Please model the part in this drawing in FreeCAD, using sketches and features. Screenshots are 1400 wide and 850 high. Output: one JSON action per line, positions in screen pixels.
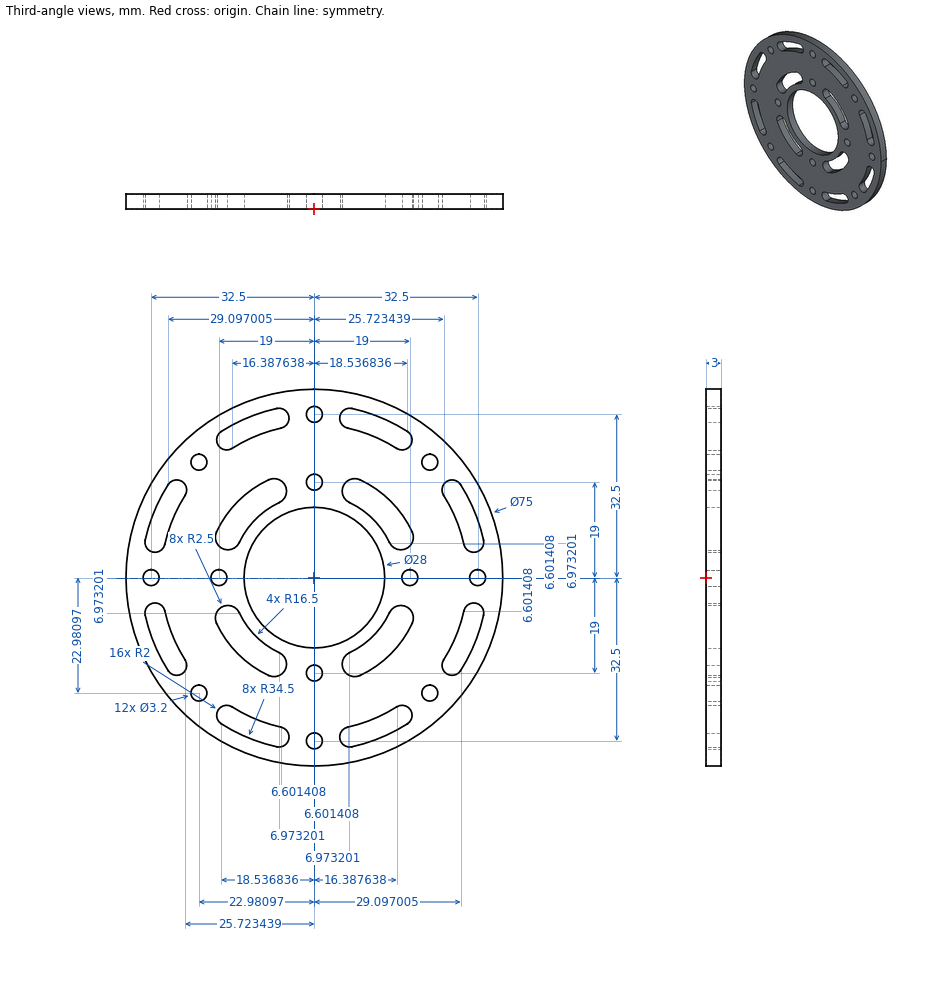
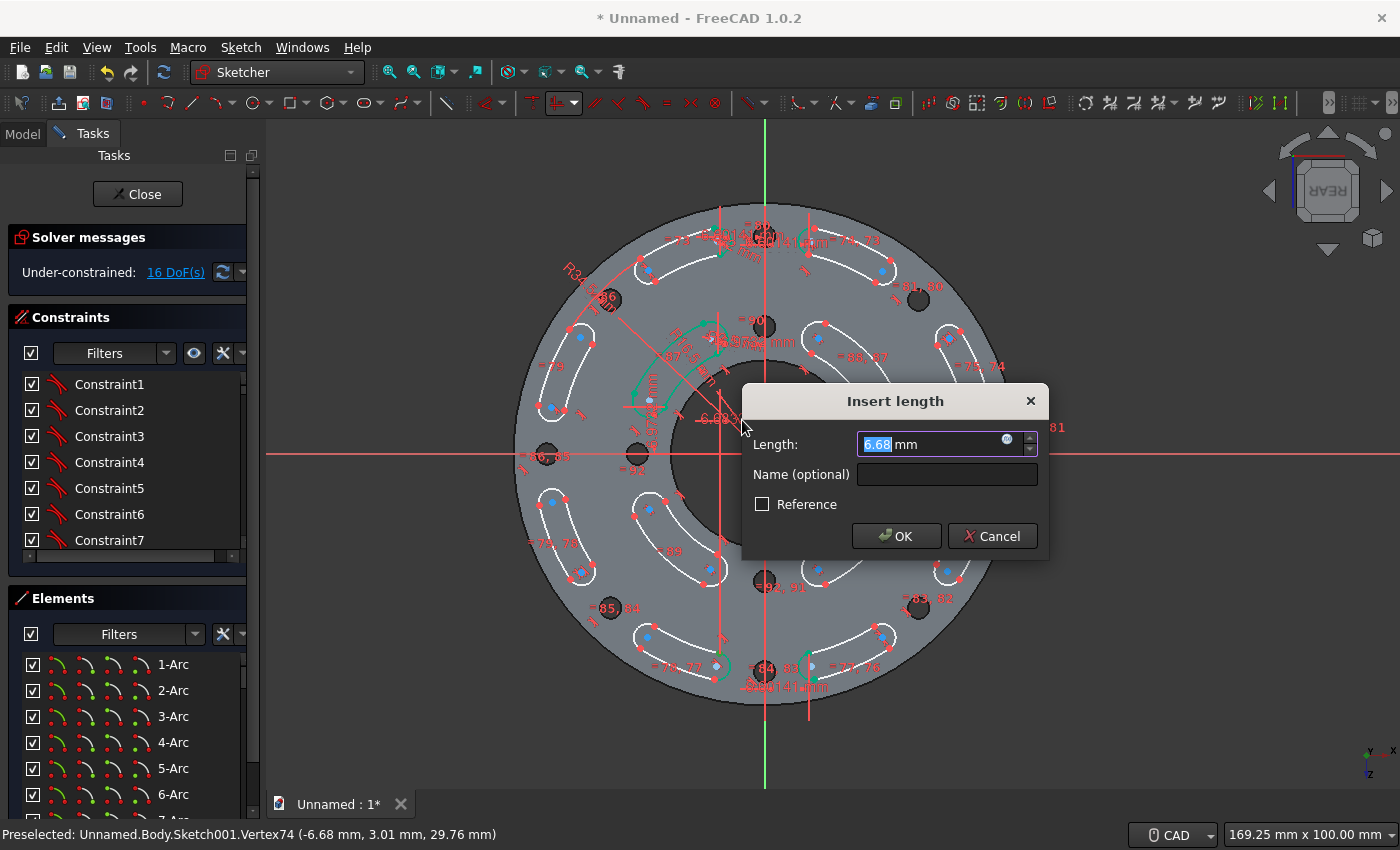
{"action": "type", "text": "6.601408"}
{"action": "key", "text": "Return"}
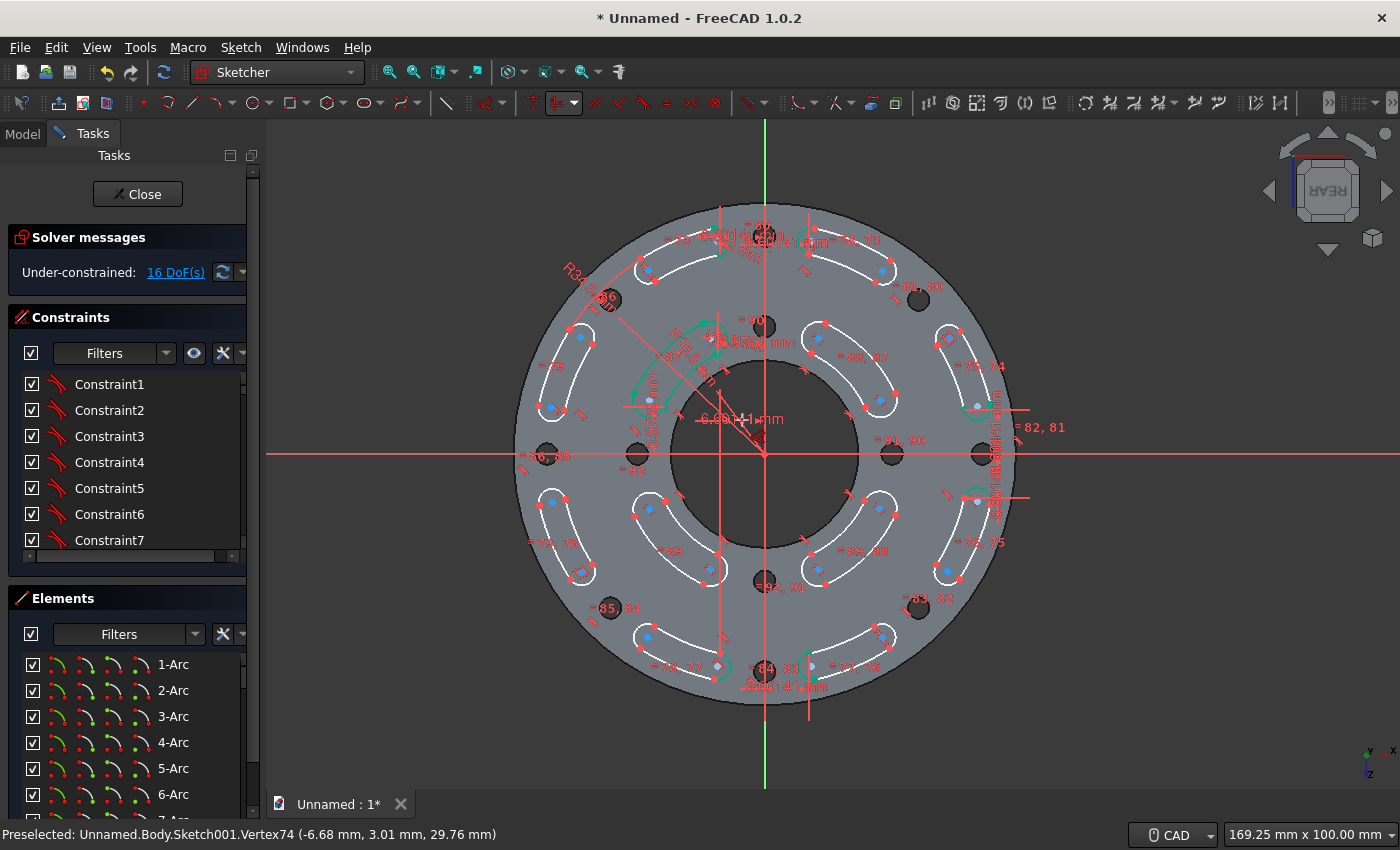
{"action": "left_click", "coordinate": [565, 499]}
{"action": "left_click", "coordinate": [531, 477]}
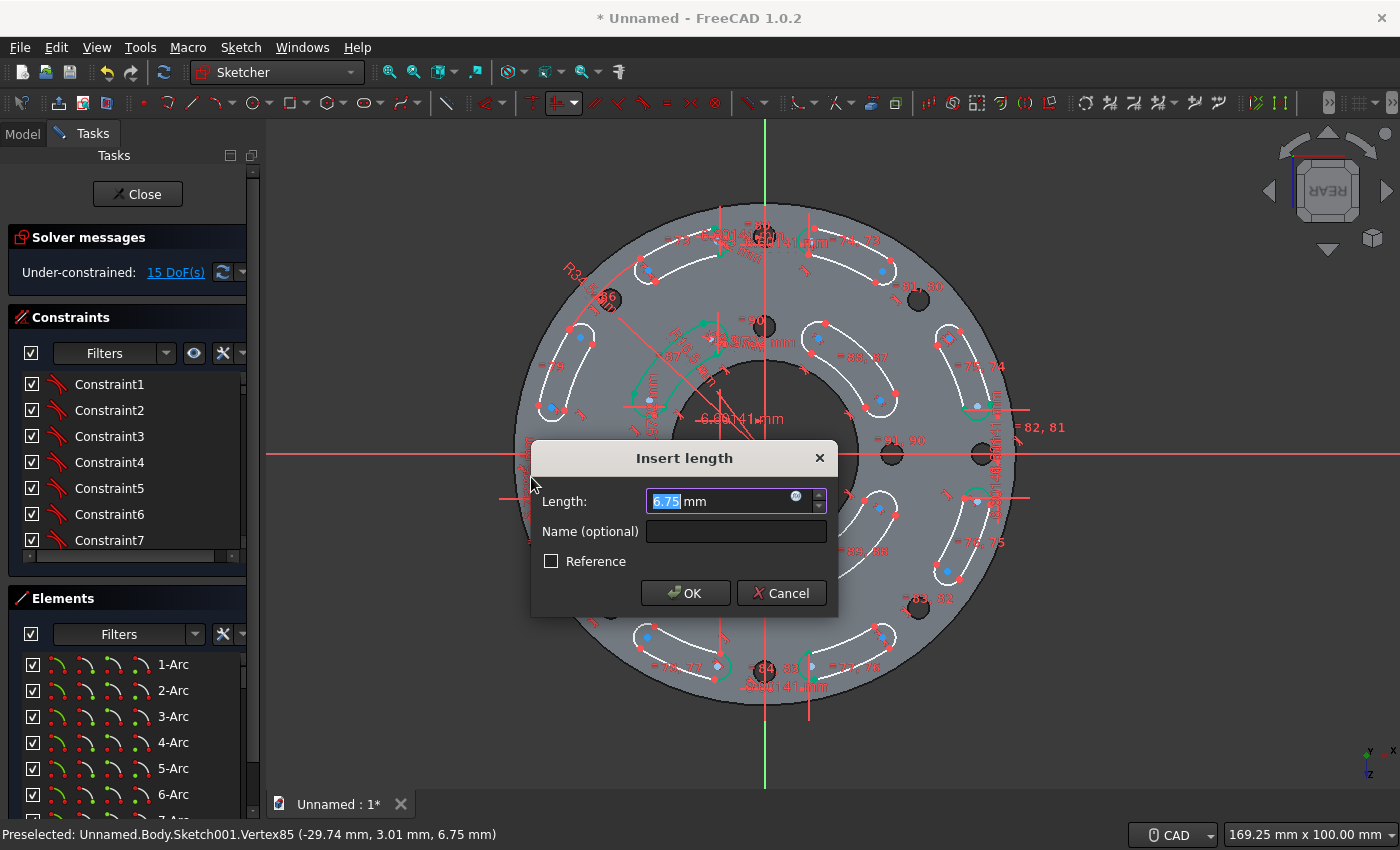
{"action": "type", "text": "6.601408"}
{"action": "key", "text": "Return"}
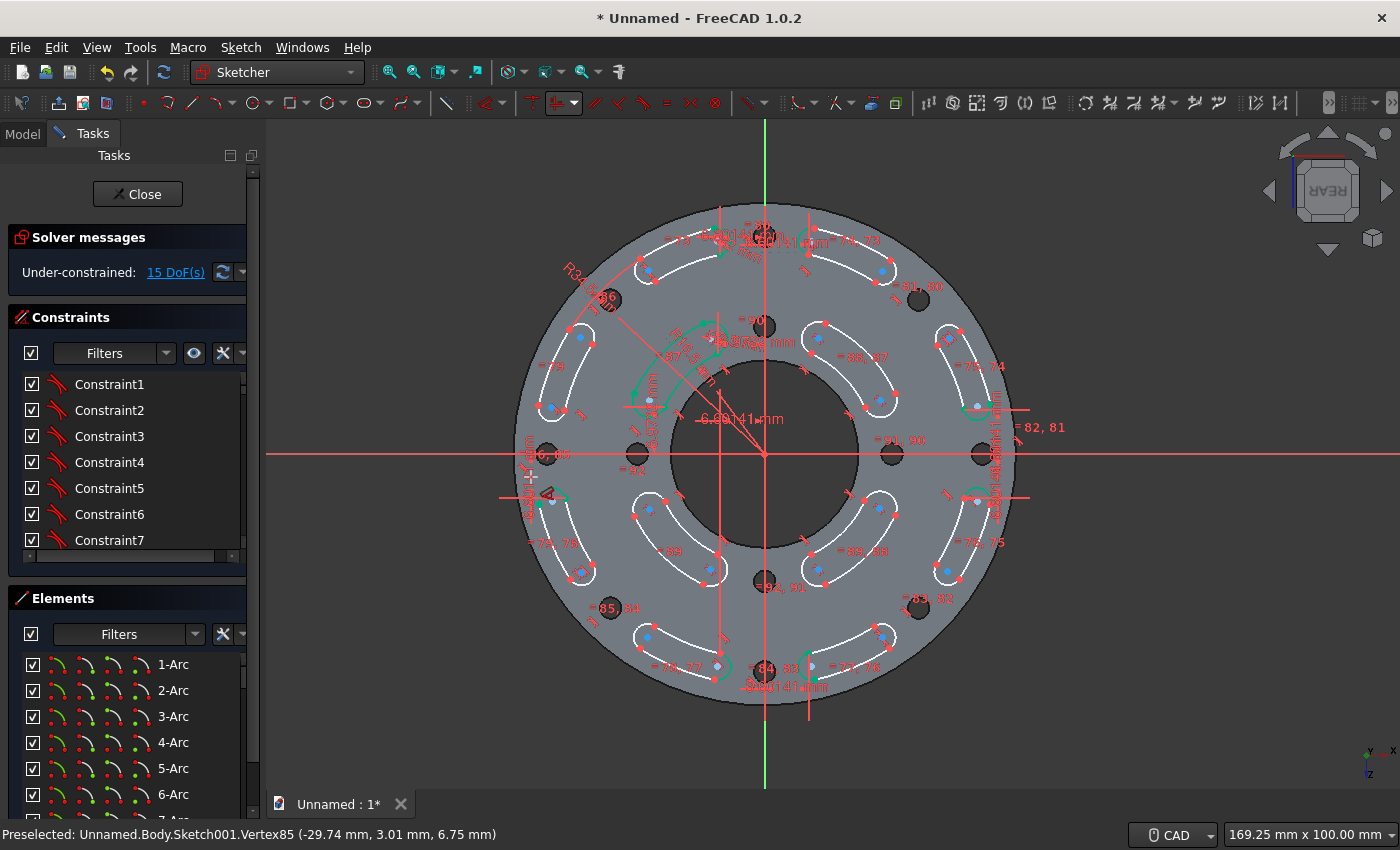
{"action": "left_click", "coordinate": [565, 411]}
{"action": "left_click", "coordinate": [531, 432]}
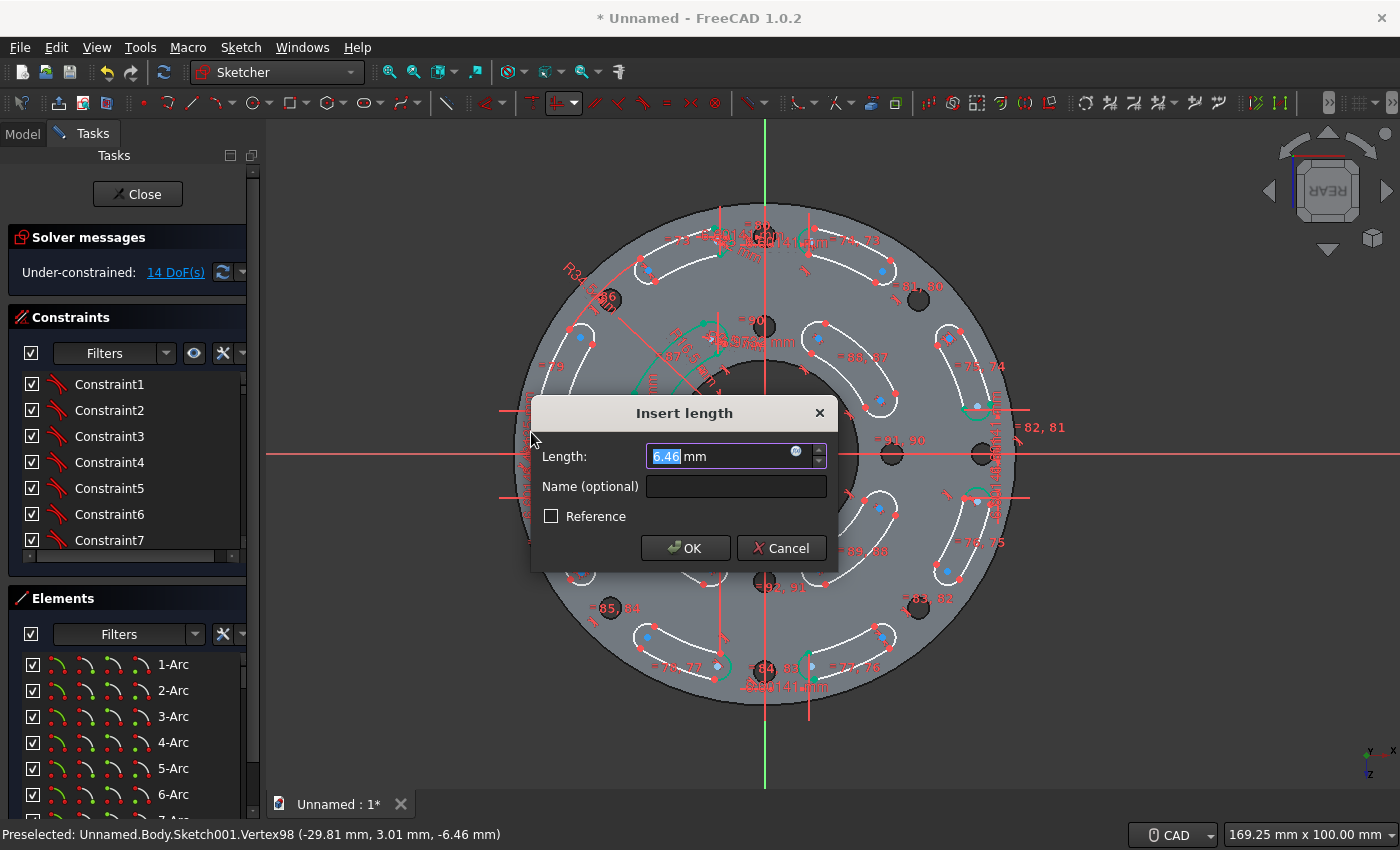
{"action": "type", "text": "6.601408"}
{"action": "key", "text": "Return"}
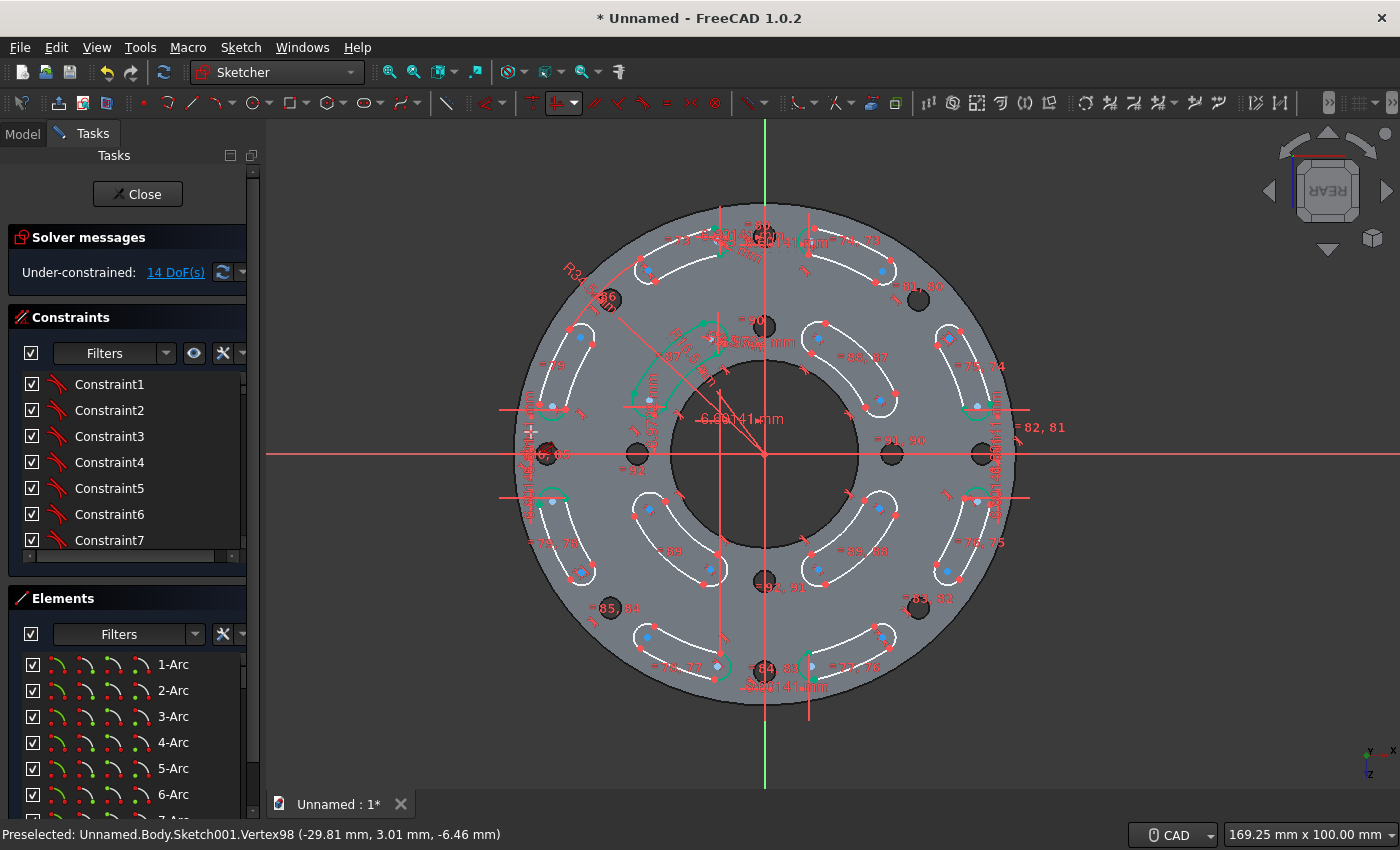
{"action": "left_click", "coordinate": [865, 408]}
{"action": "left_click", "coordinate": [899, 431]}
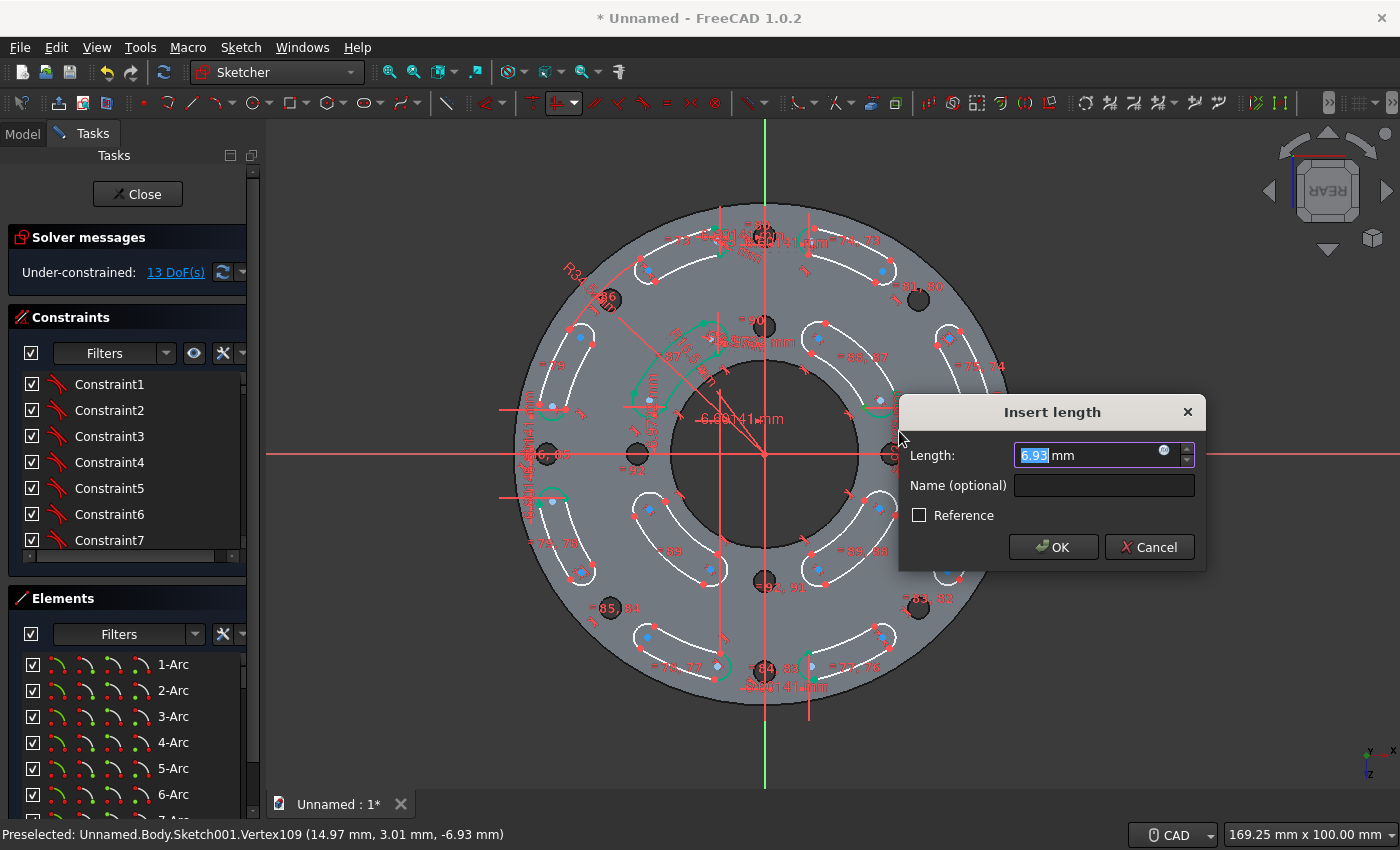
{"action": "type", "text": "6.973201"}
{"action": "key", "text": "Return"}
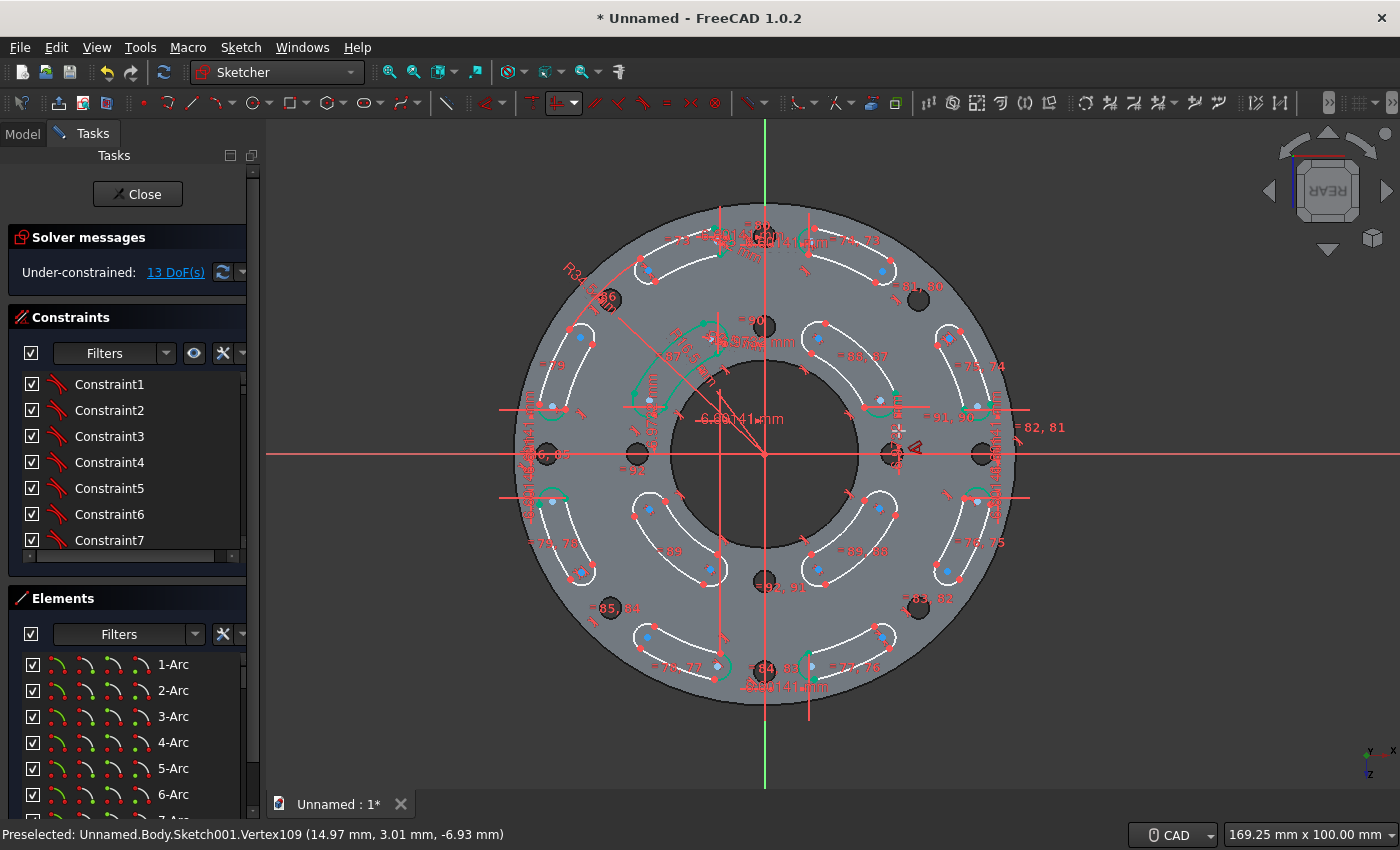
{"action": "left_click", "coordinate": [811, 354]}
{"action": "left_click", "coordinate": [788, 320]}